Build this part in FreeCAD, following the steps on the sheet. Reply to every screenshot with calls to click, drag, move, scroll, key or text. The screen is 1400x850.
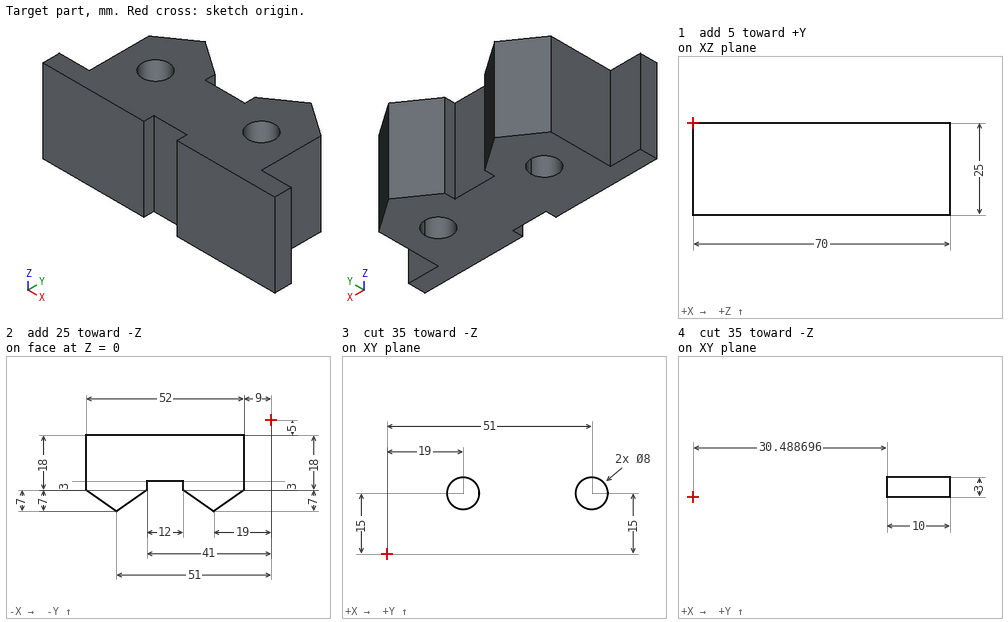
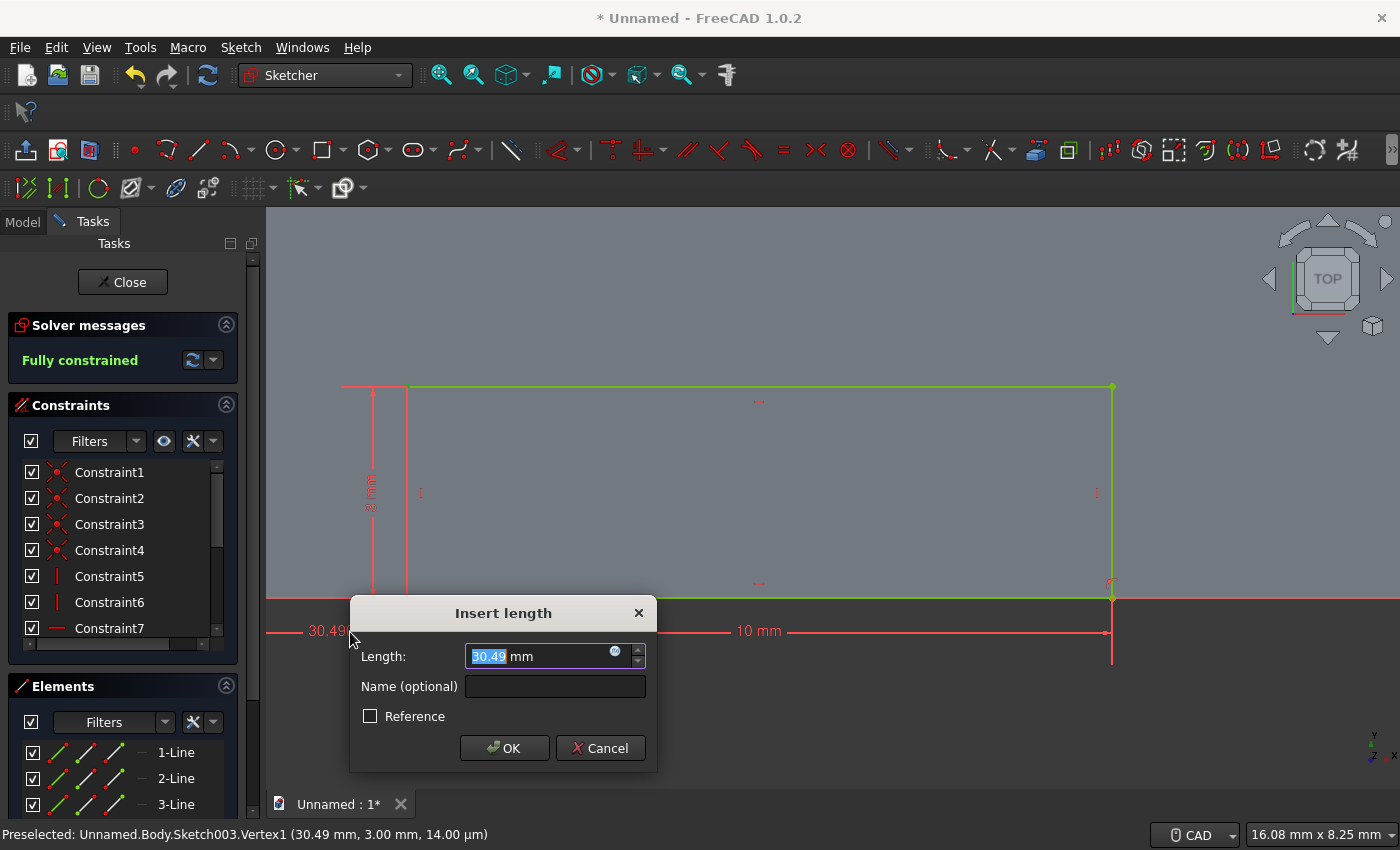
text(30.488696)
key(Return)
key(Escape)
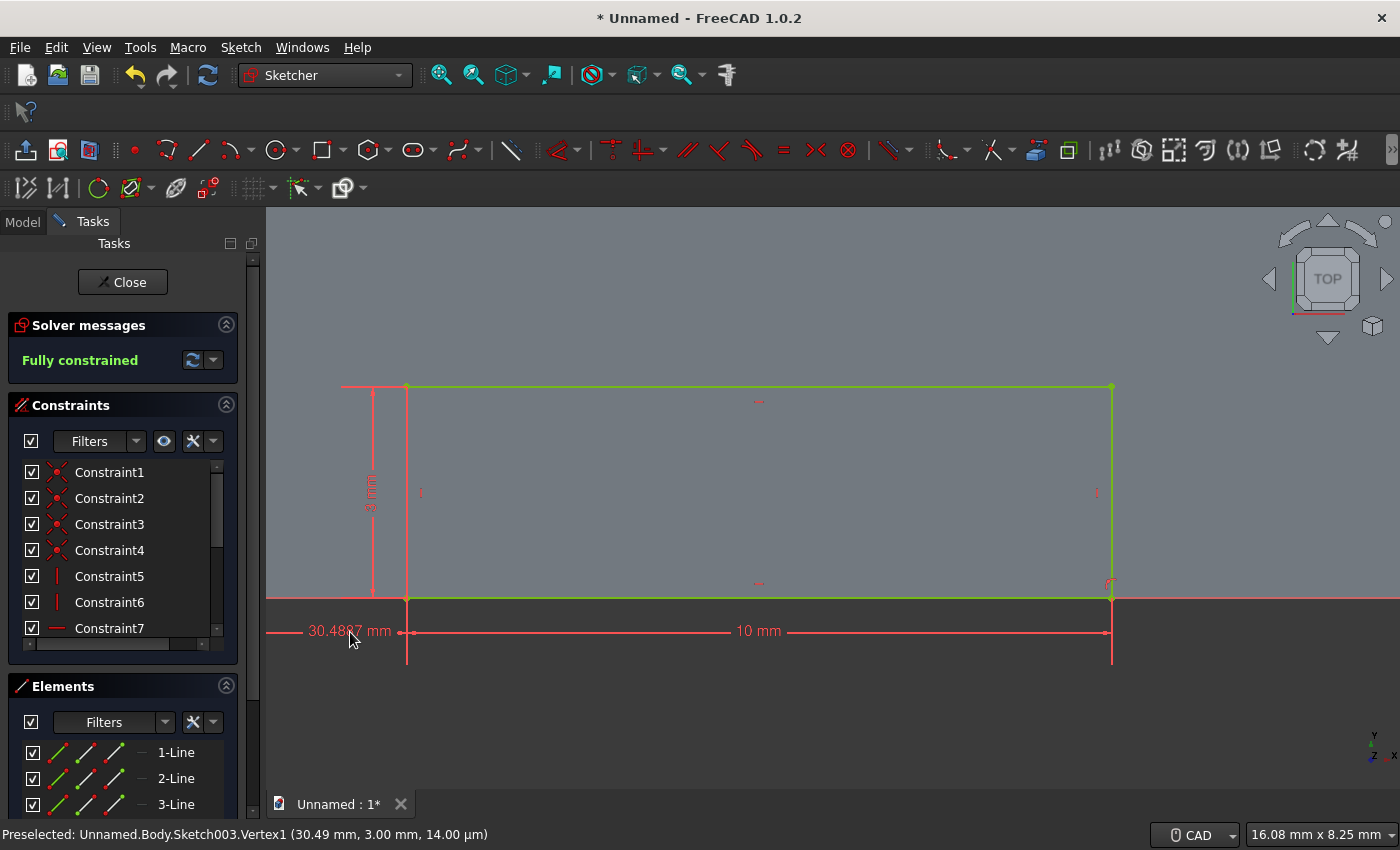
click(123, 282)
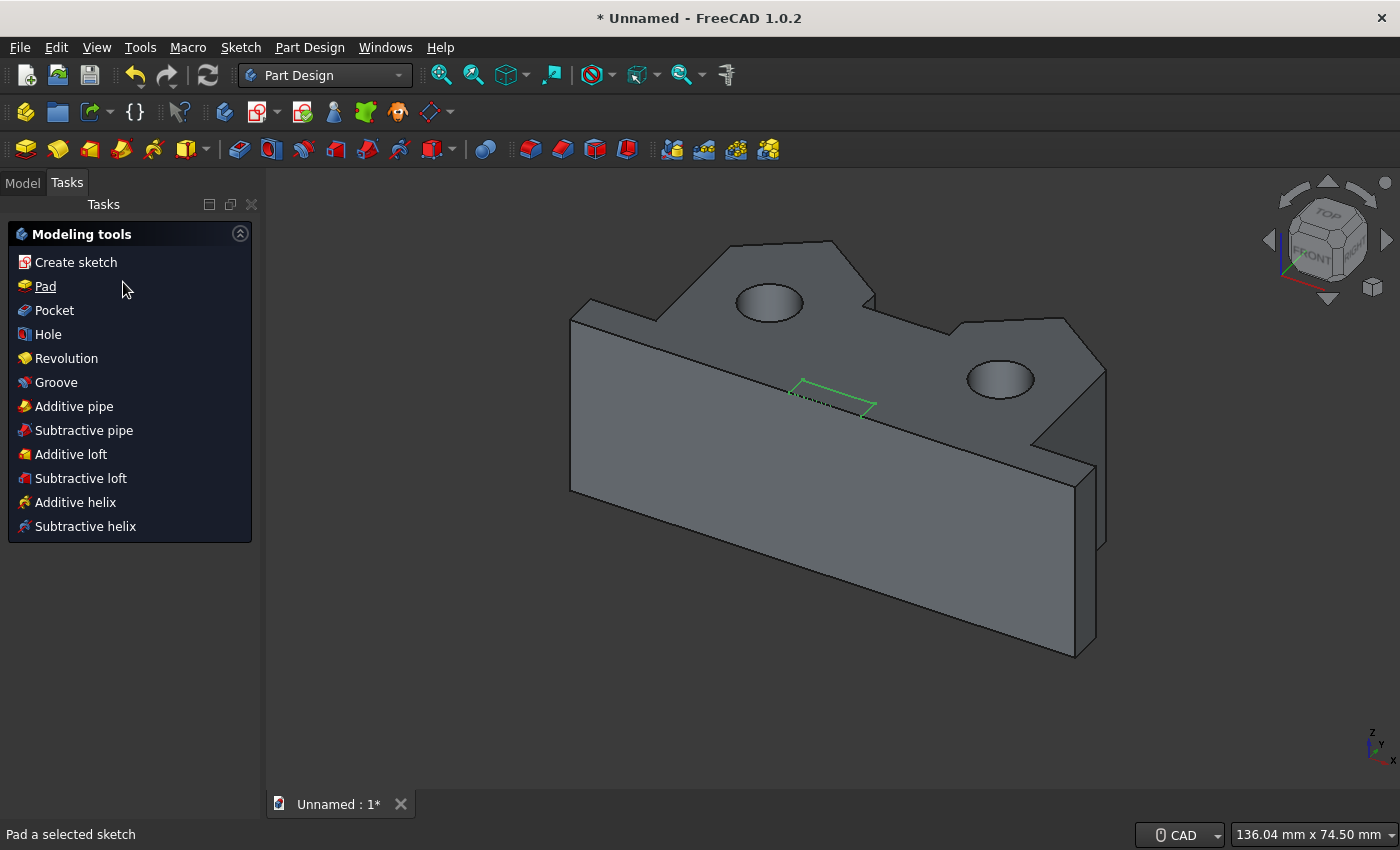
click(240, 150)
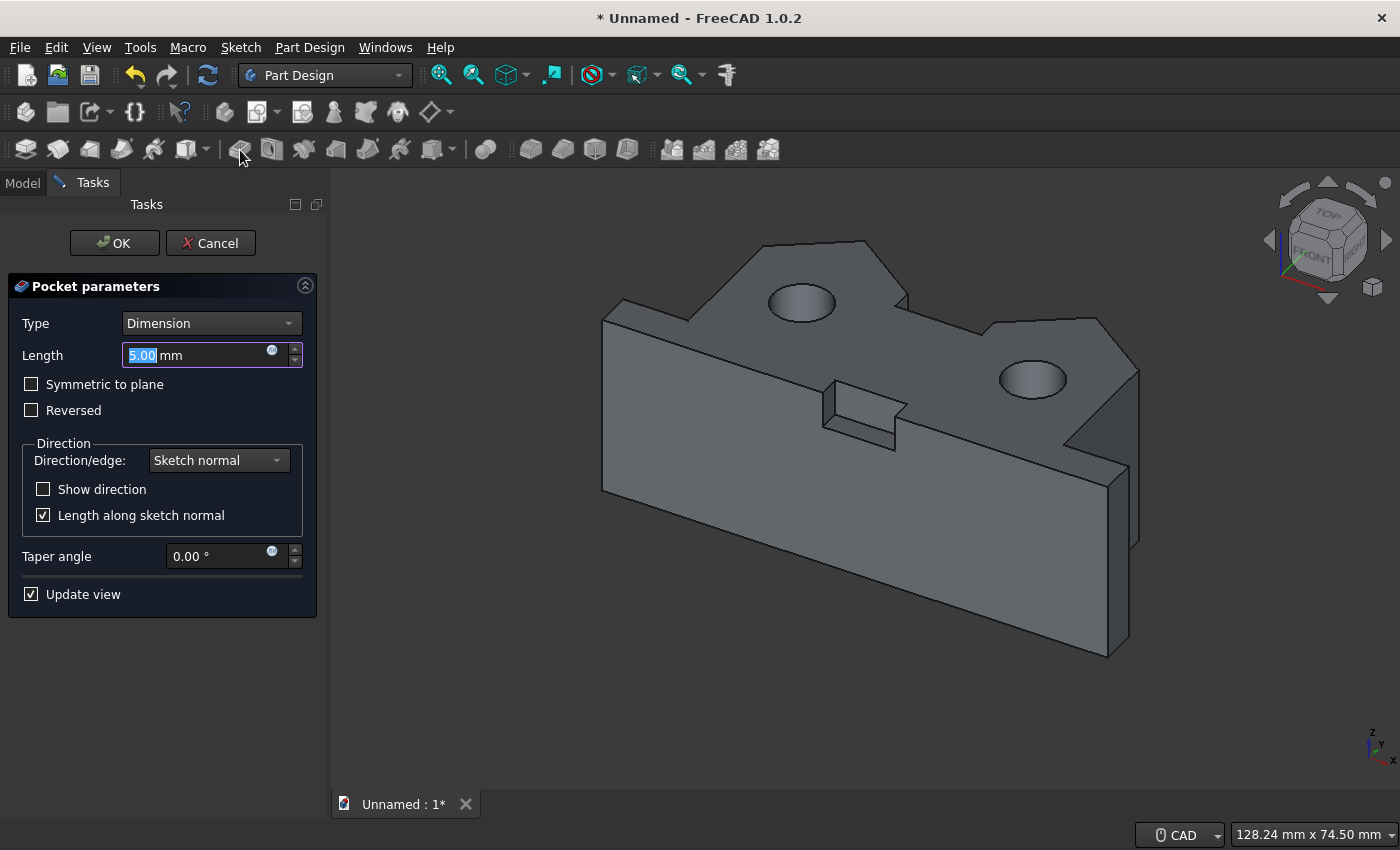
text(35)
key(Tab)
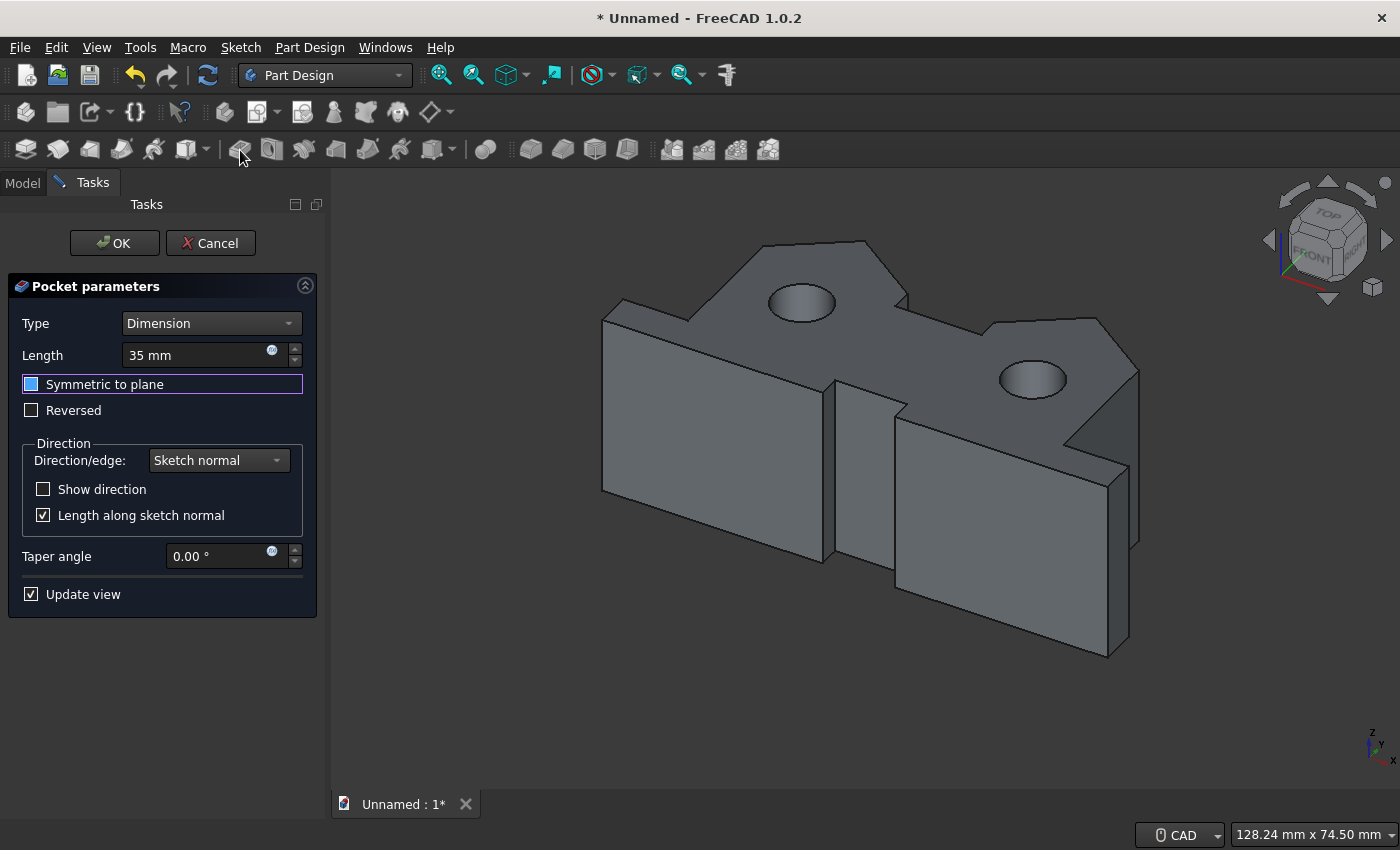
click(115, 243)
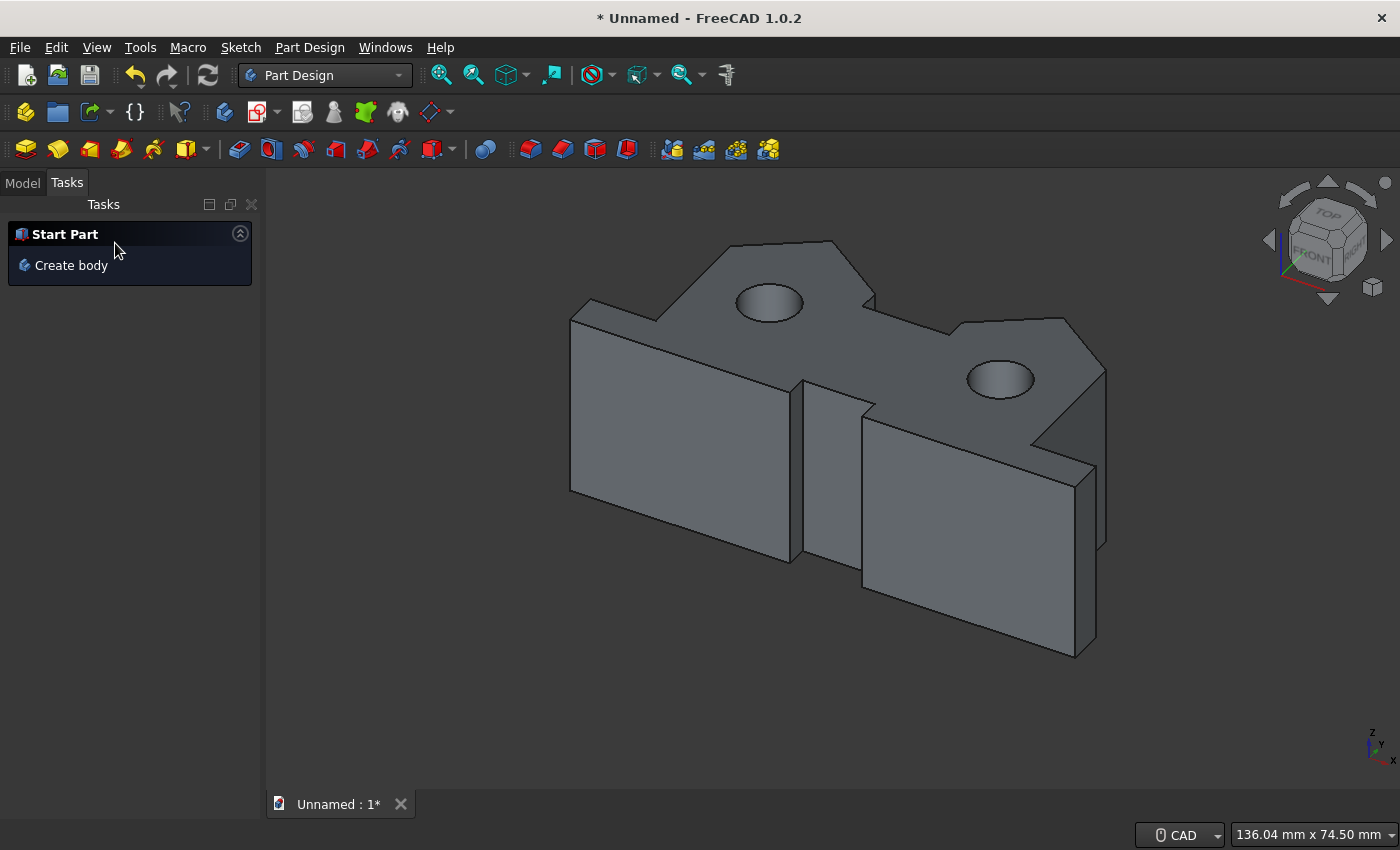
key(0)